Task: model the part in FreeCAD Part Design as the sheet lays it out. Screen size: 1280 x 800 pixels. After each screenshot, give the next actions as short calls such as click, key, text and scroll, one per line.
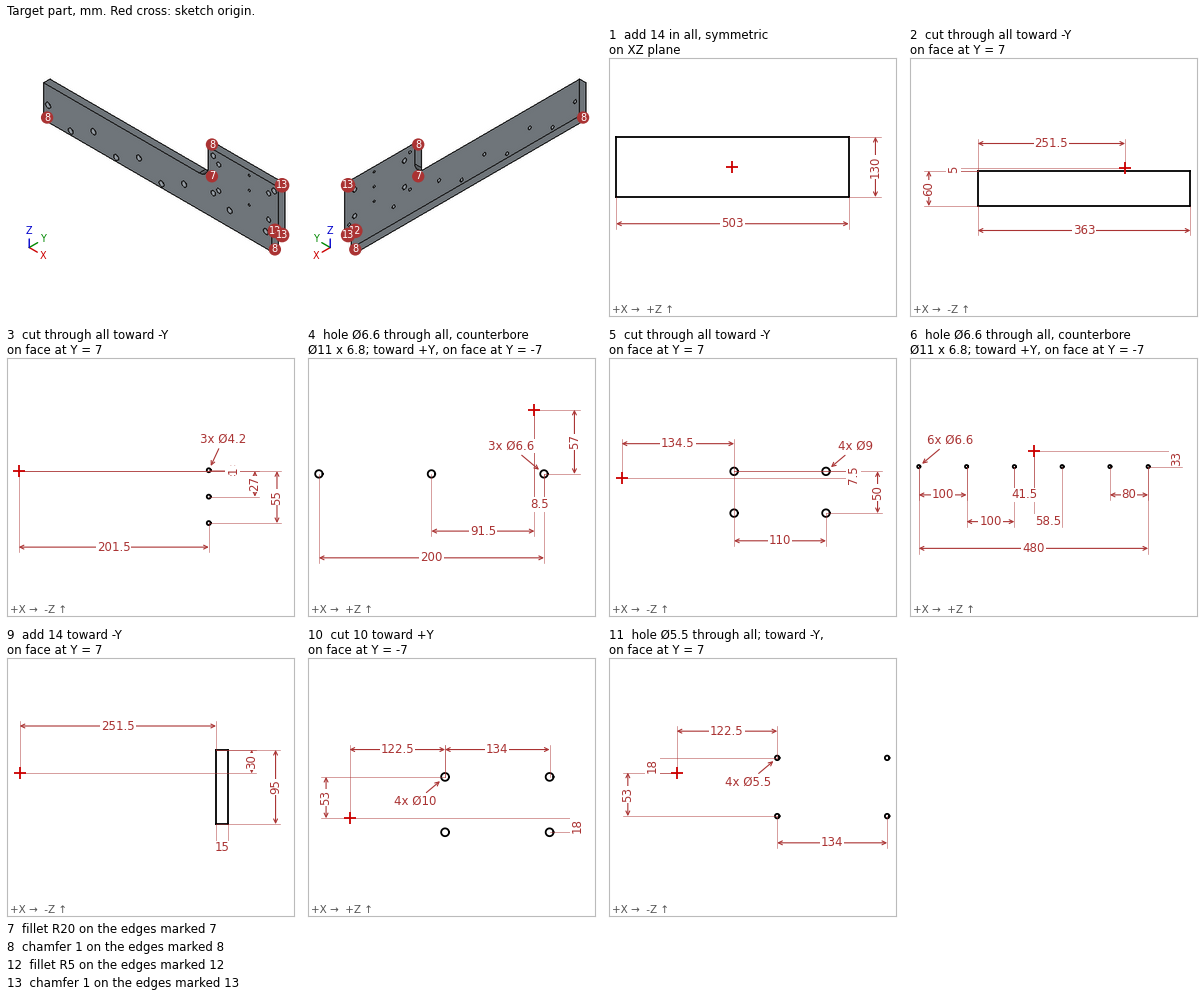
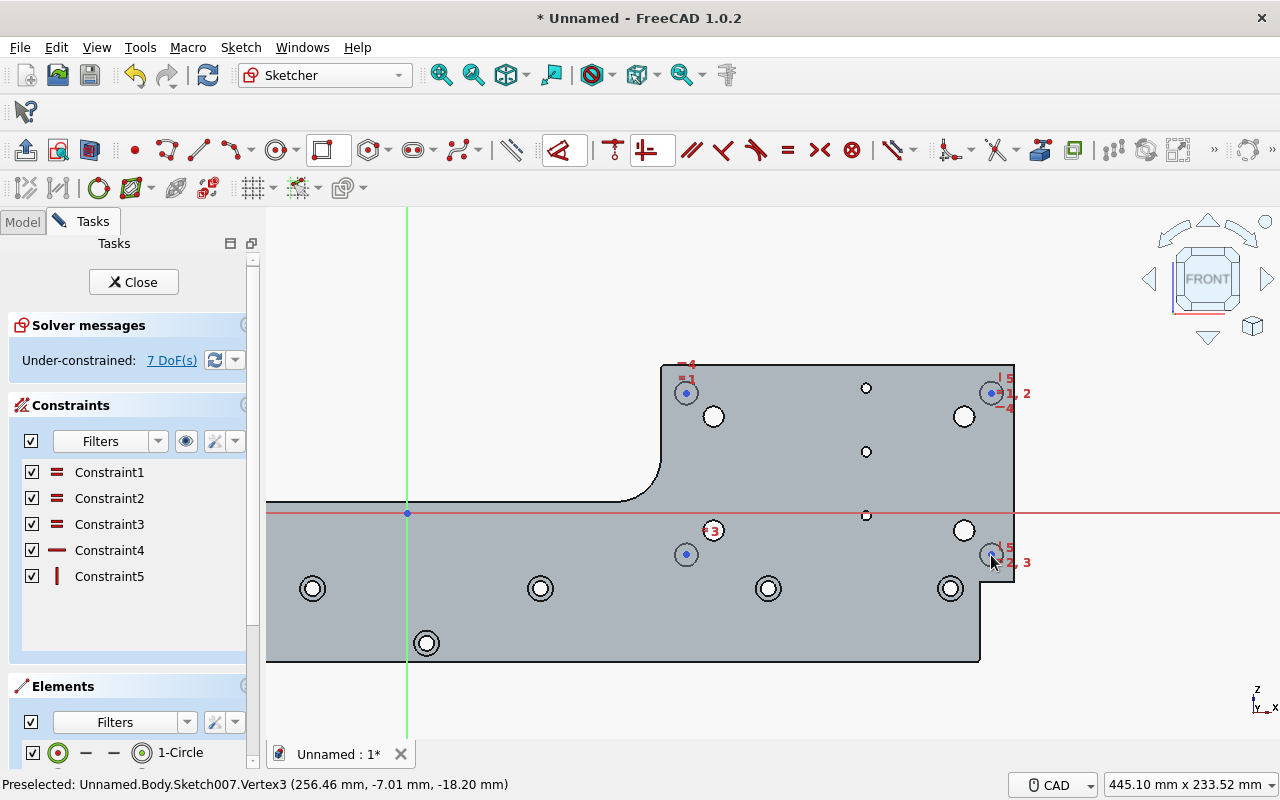
click(686, 393)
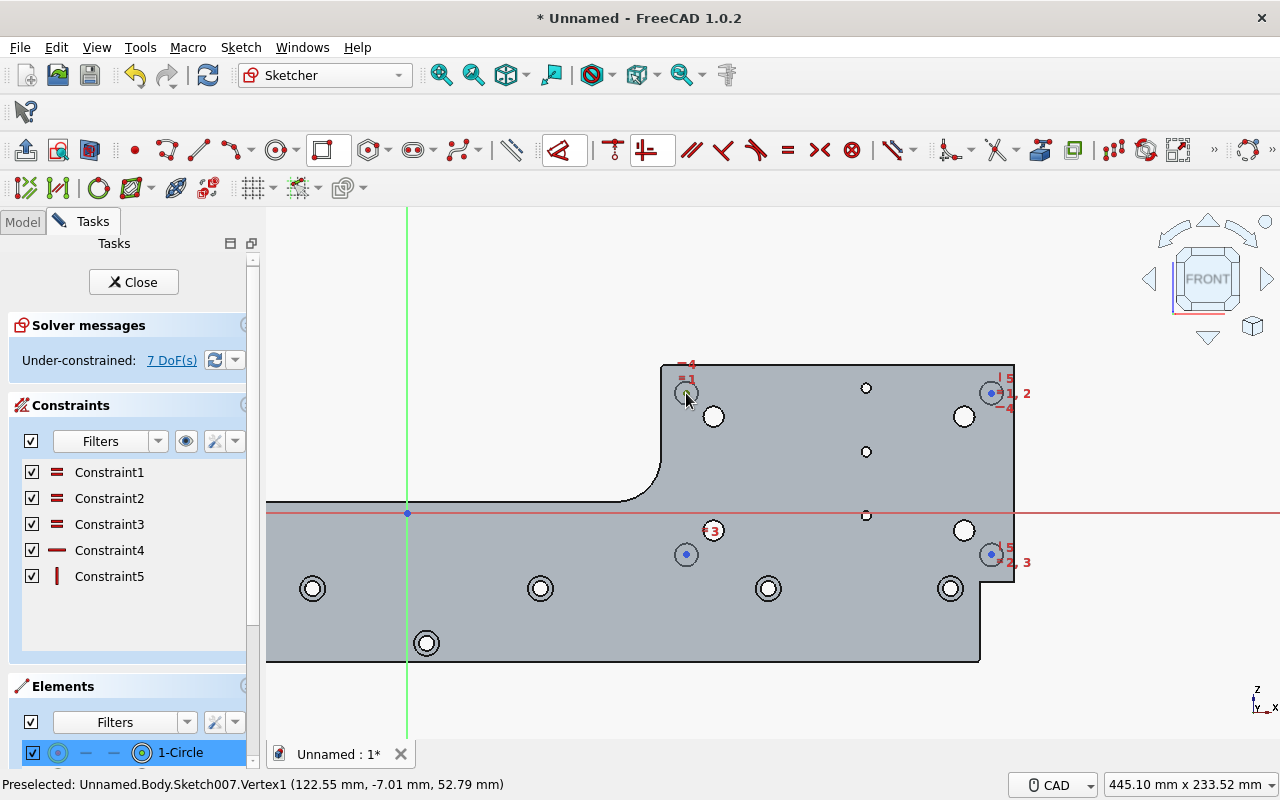
click(686, 555)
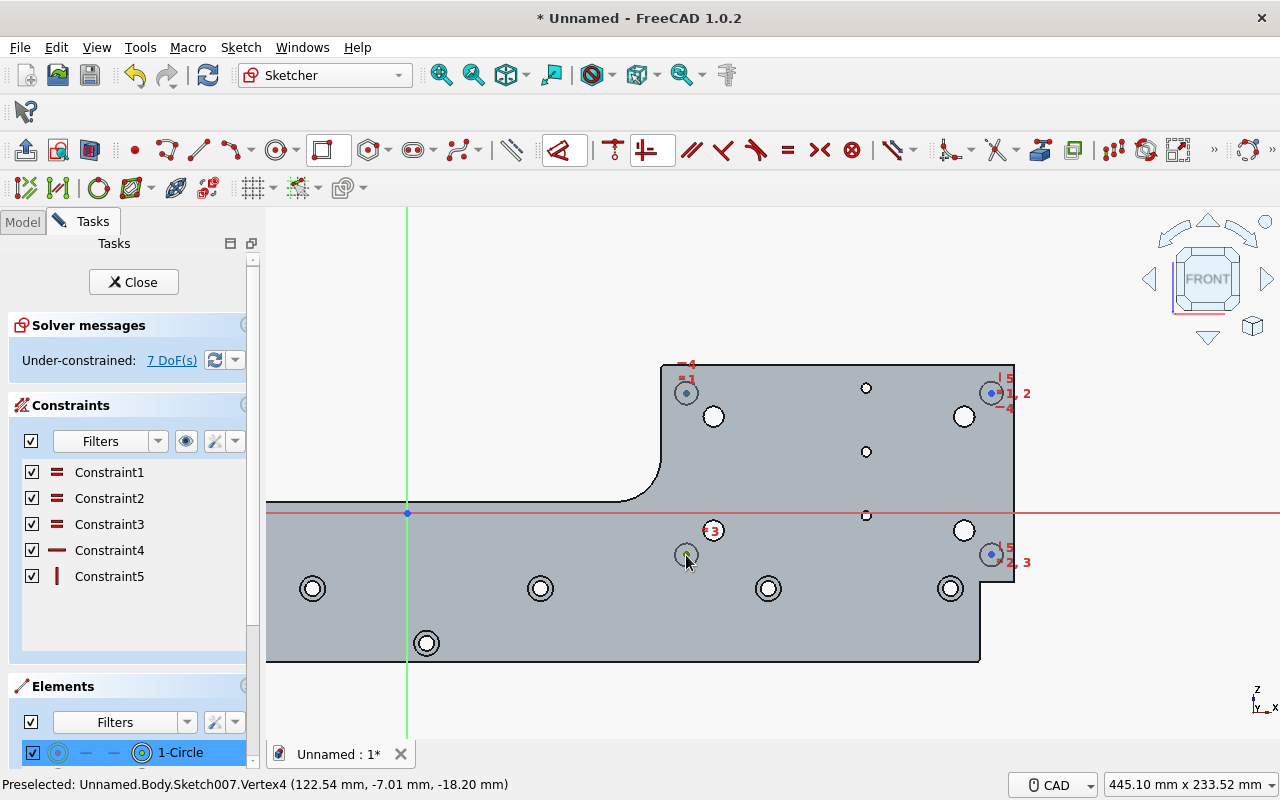
key(v)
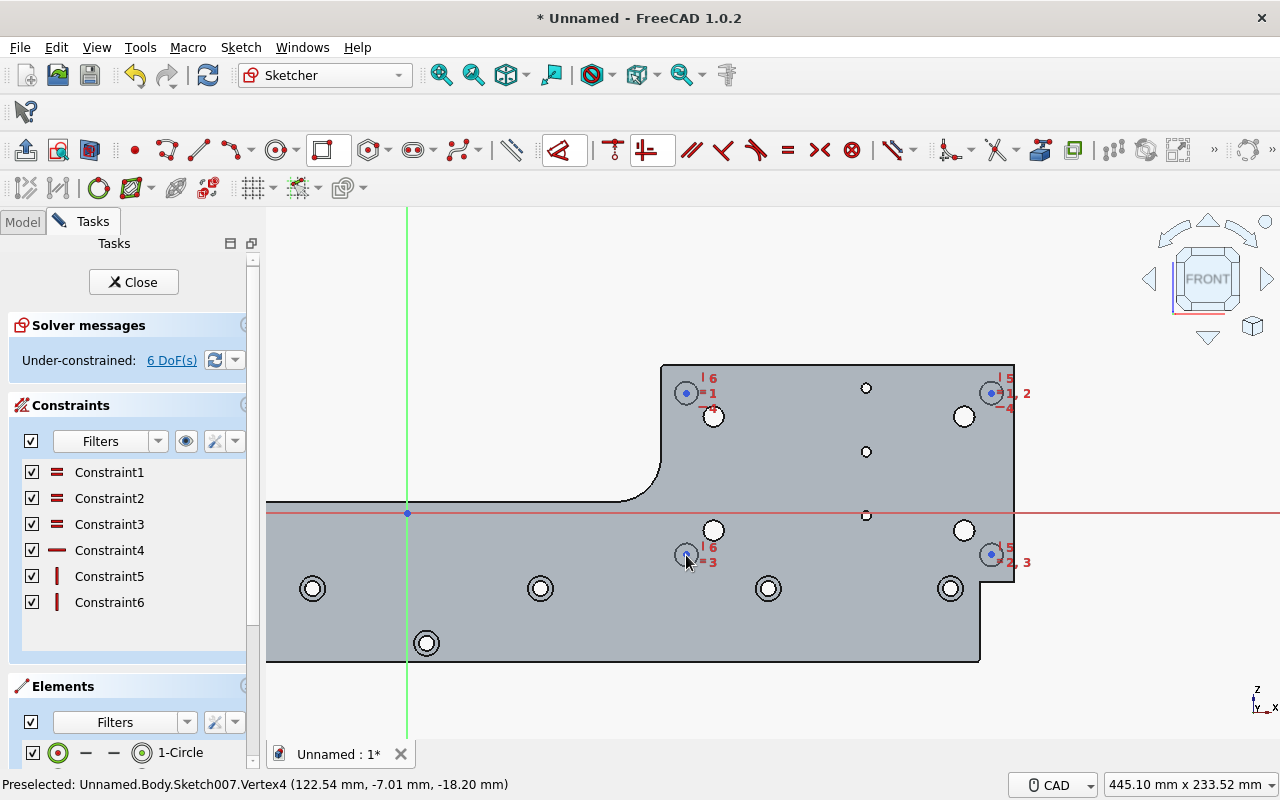
click(991, 555)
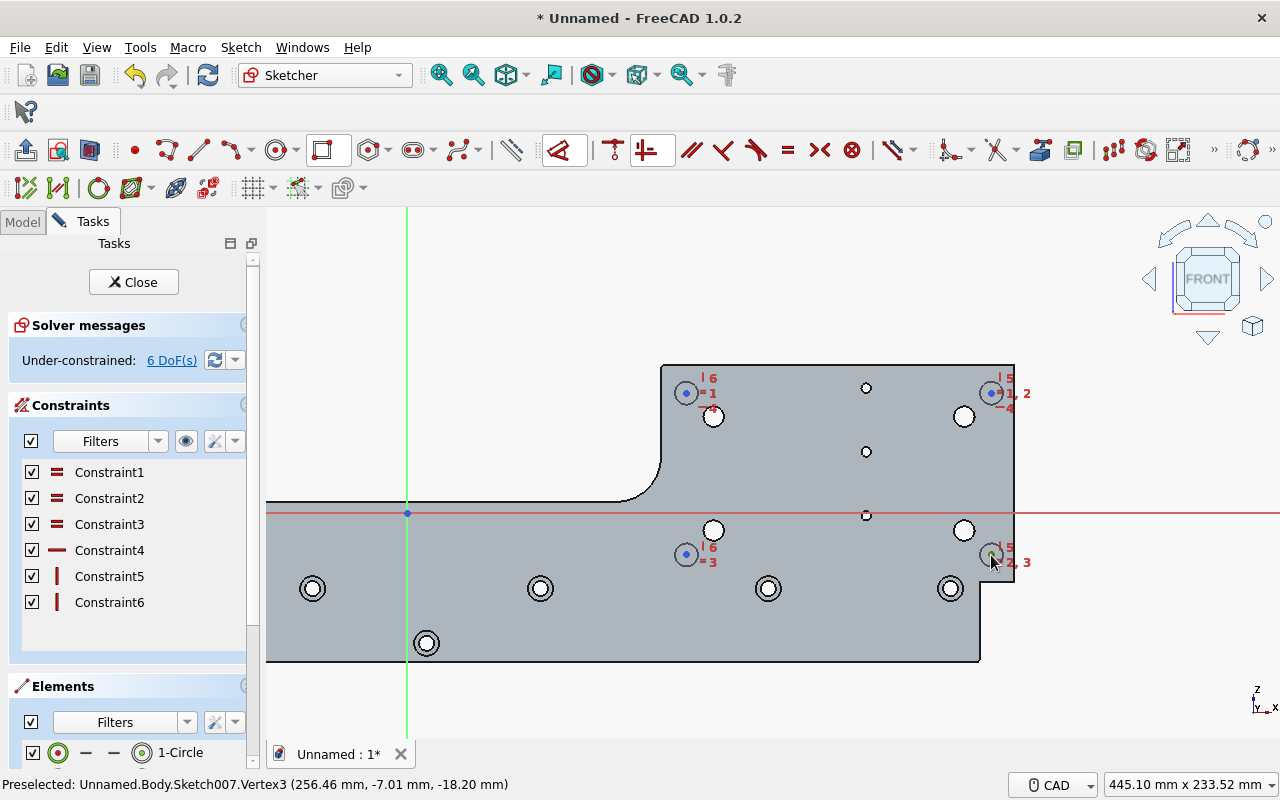
click(686, 555)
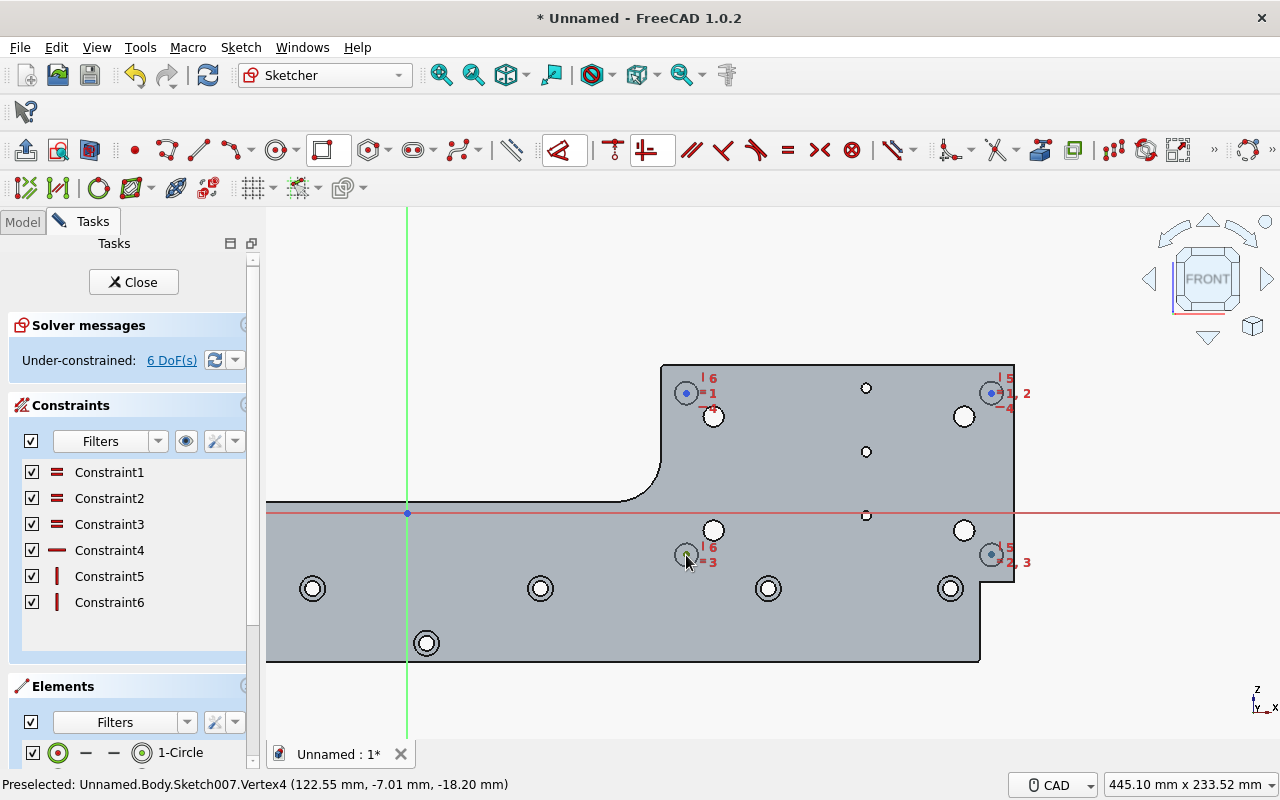
key(h)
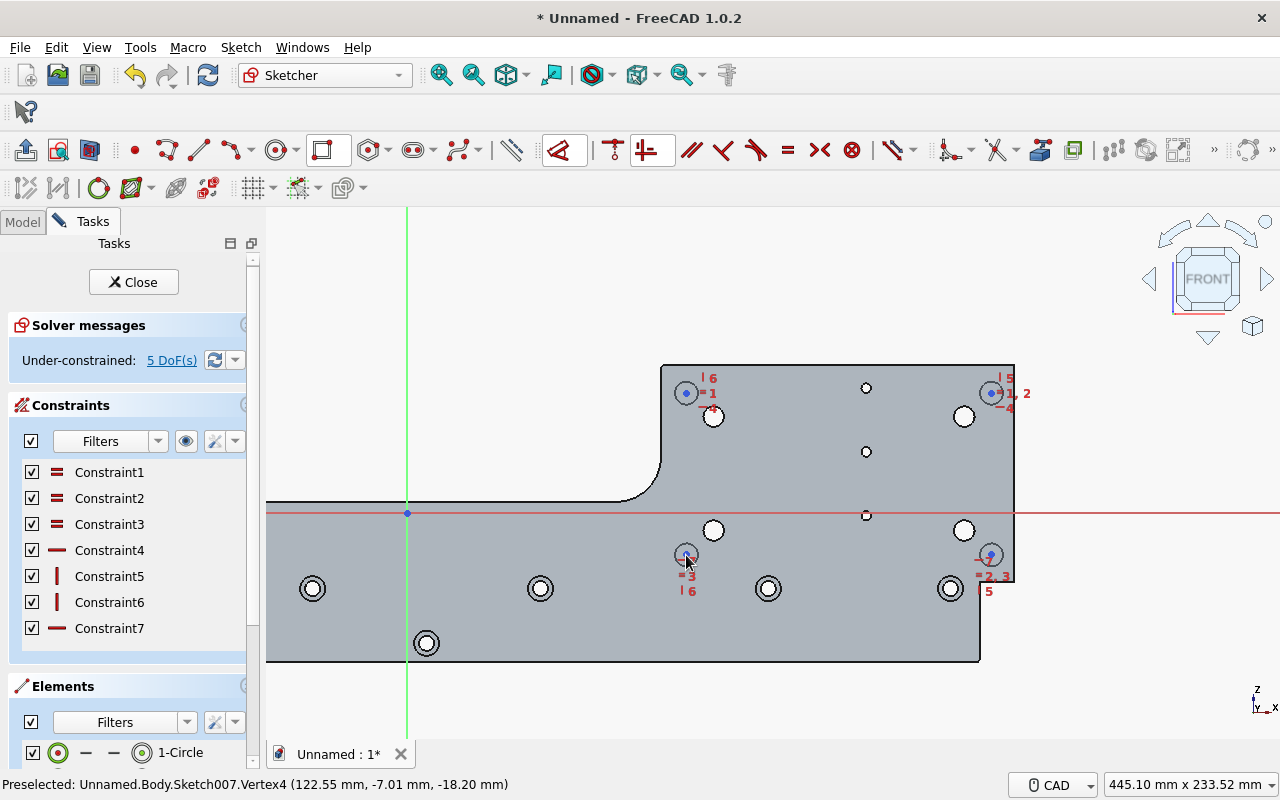
scroll(694, 385, up, 3)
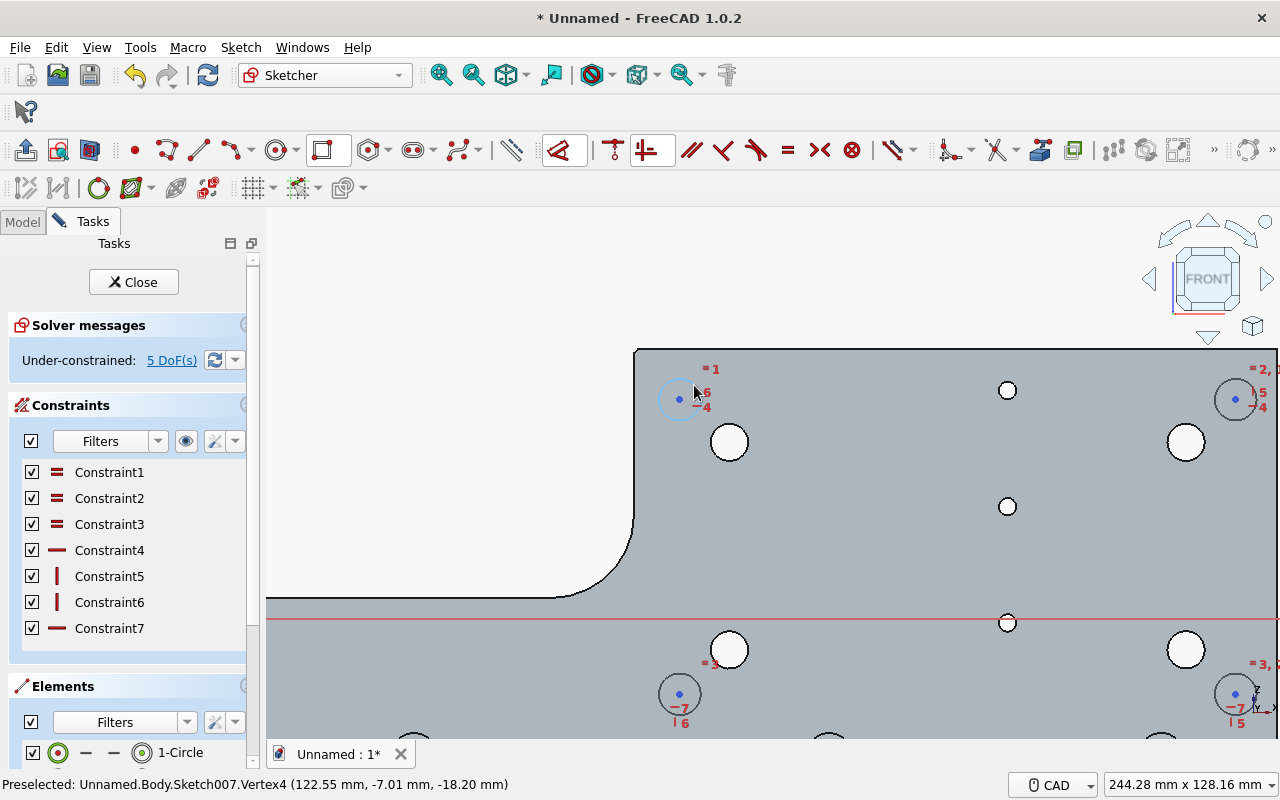
click(665, 385)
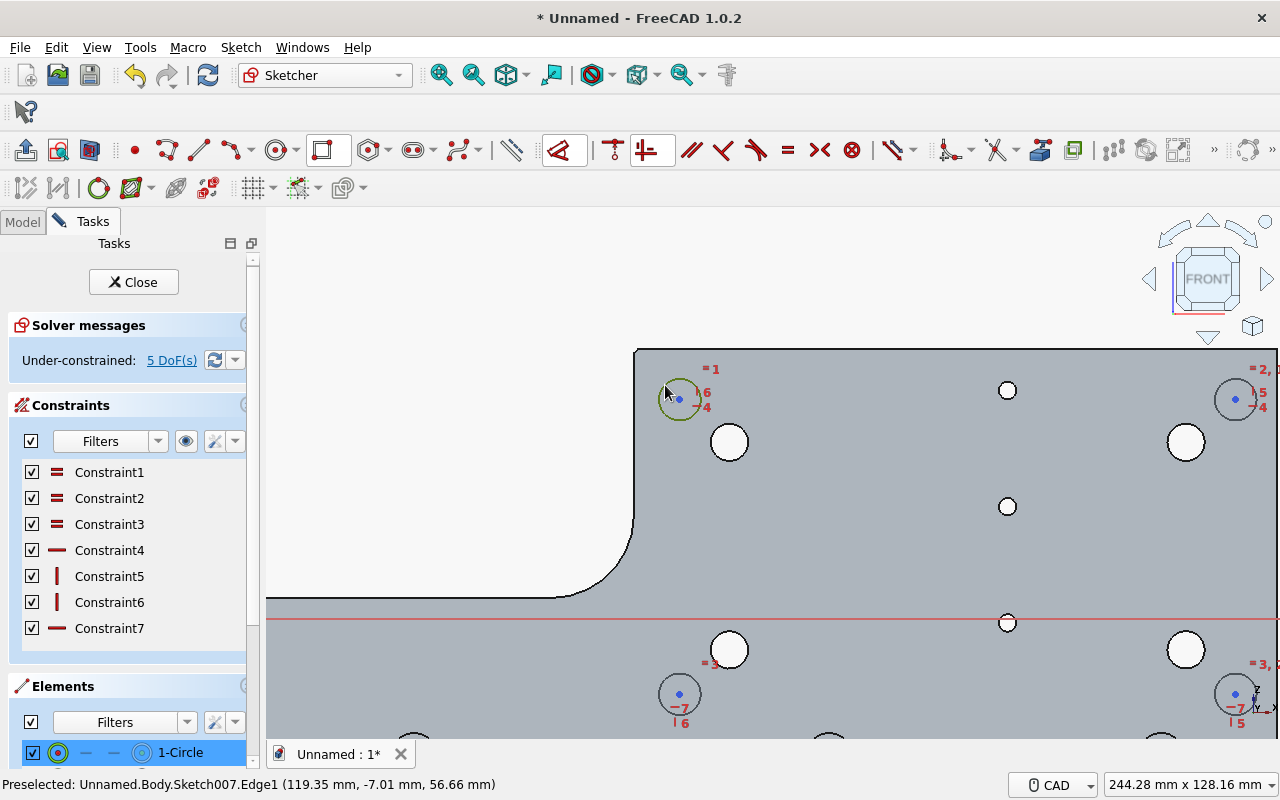
key(k)
key(o)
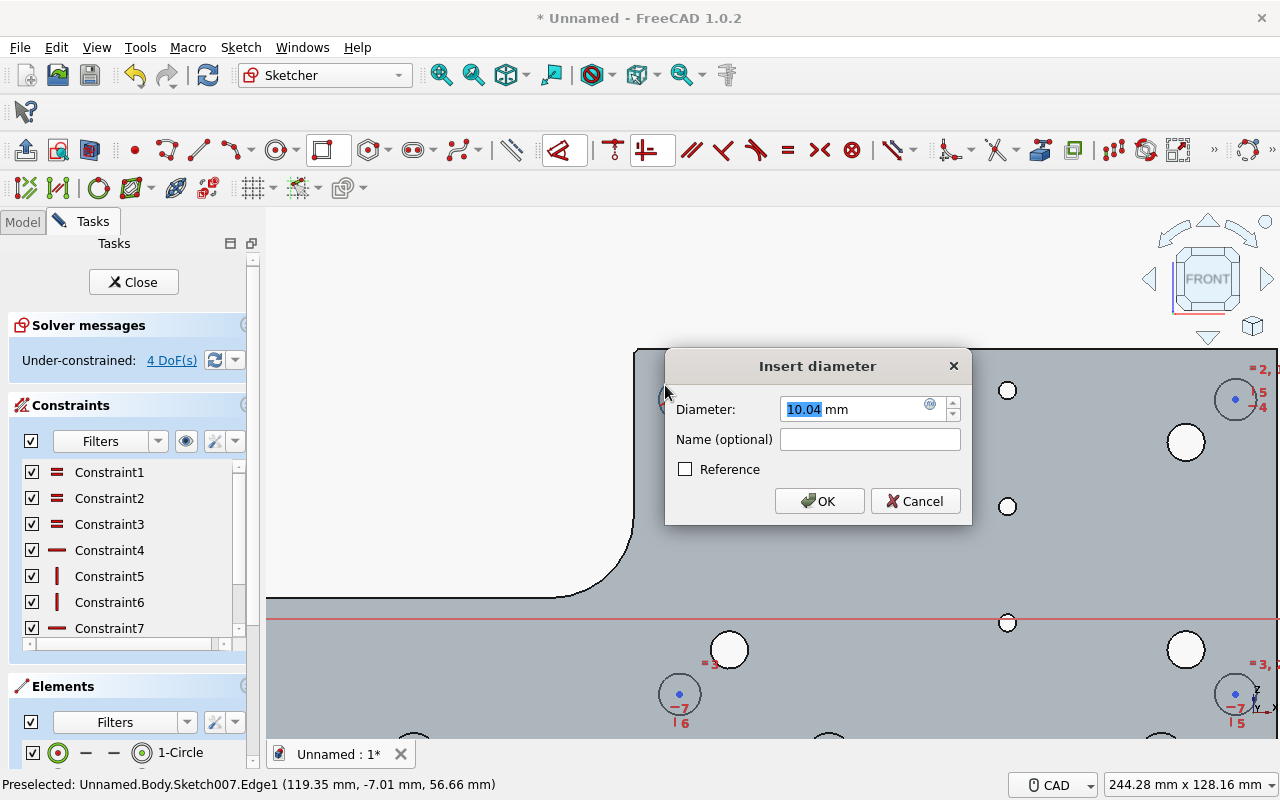
text(10)
key(Return)